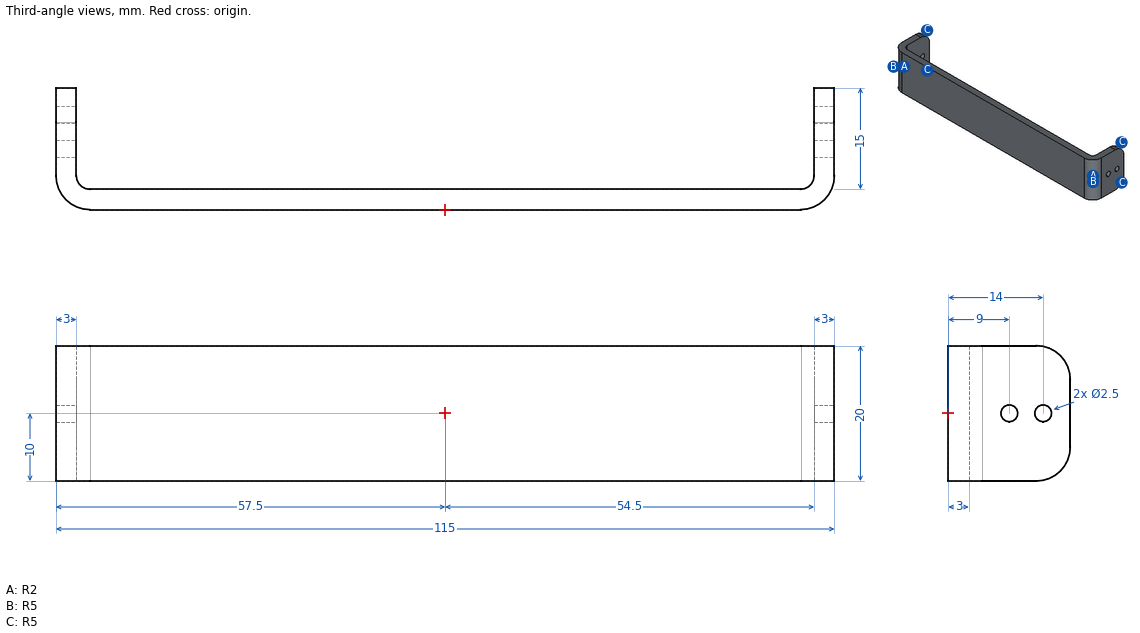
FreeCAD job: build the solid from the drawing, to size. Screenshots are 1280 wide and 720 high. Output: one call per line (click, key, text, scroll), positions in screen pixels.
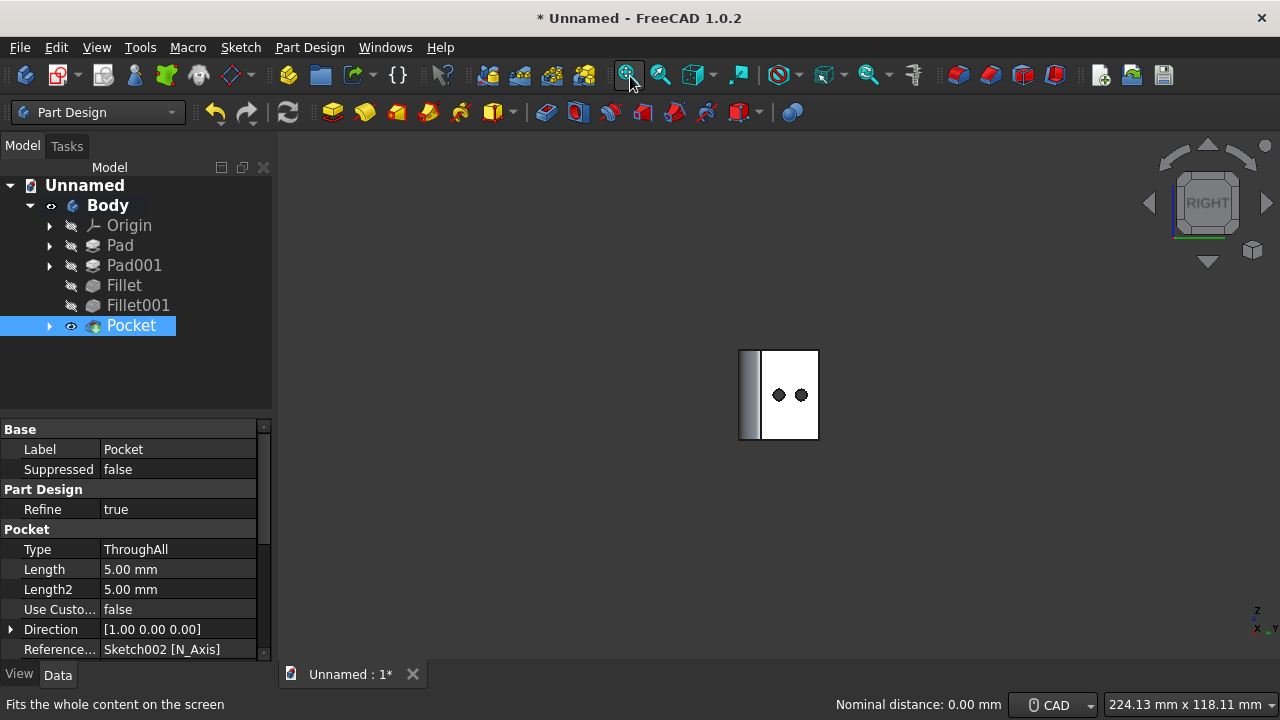
click(630, 76)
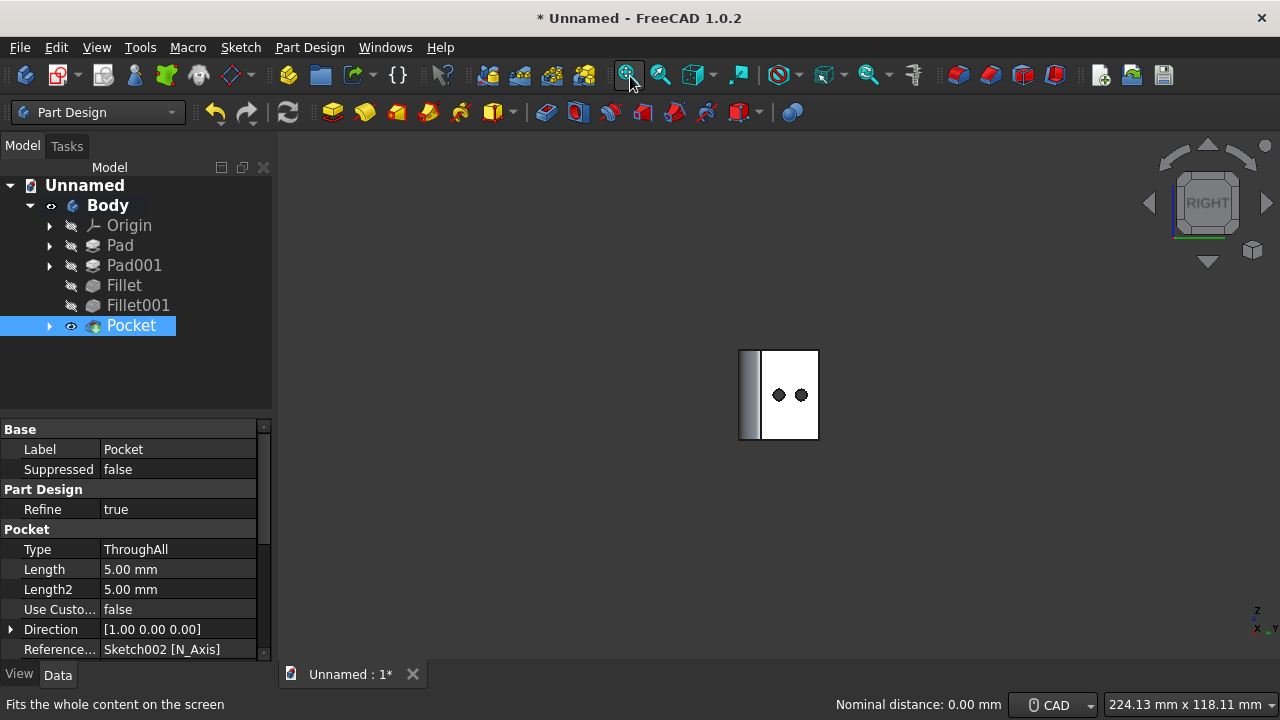
scroll(819, 439, up, 6)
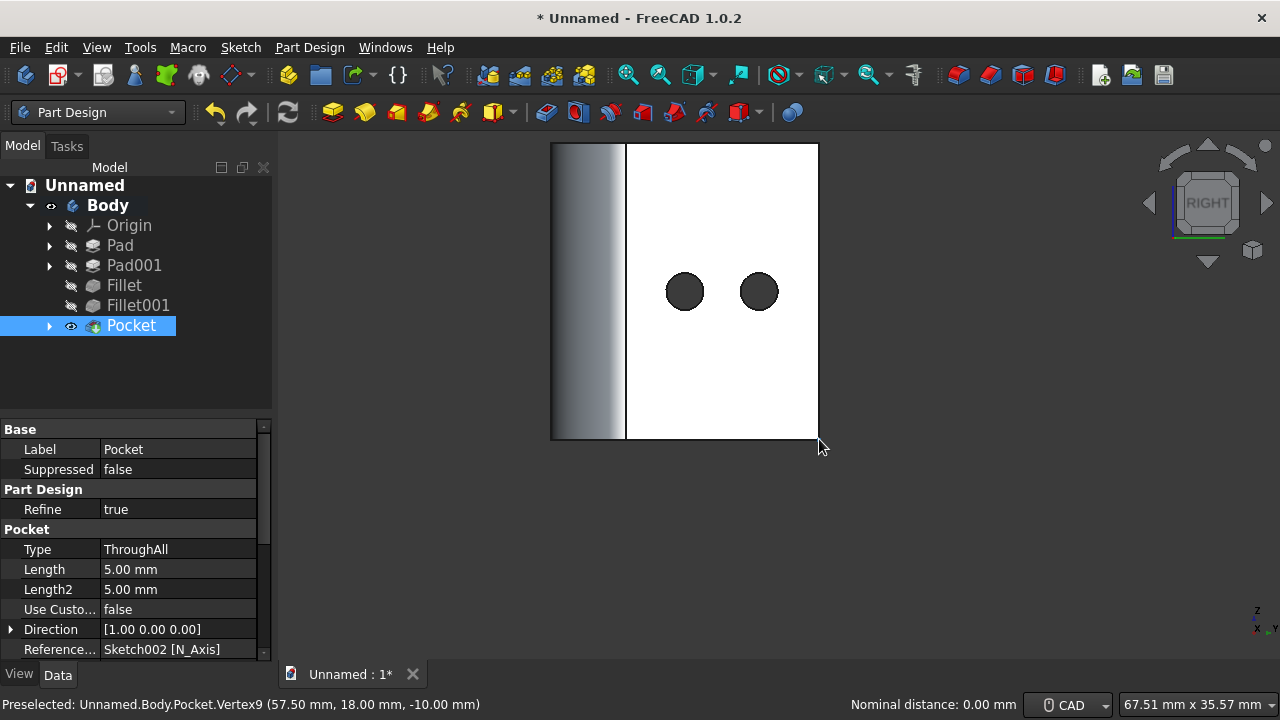
click(630, 76)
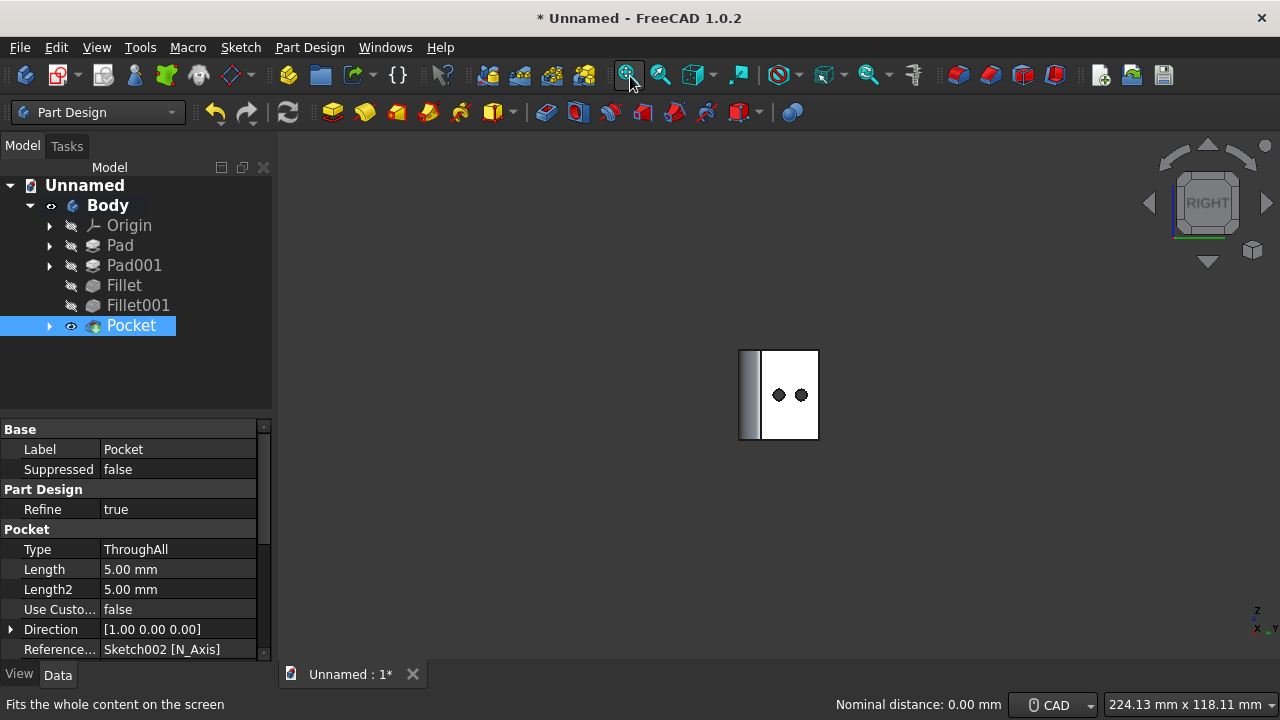
key(5)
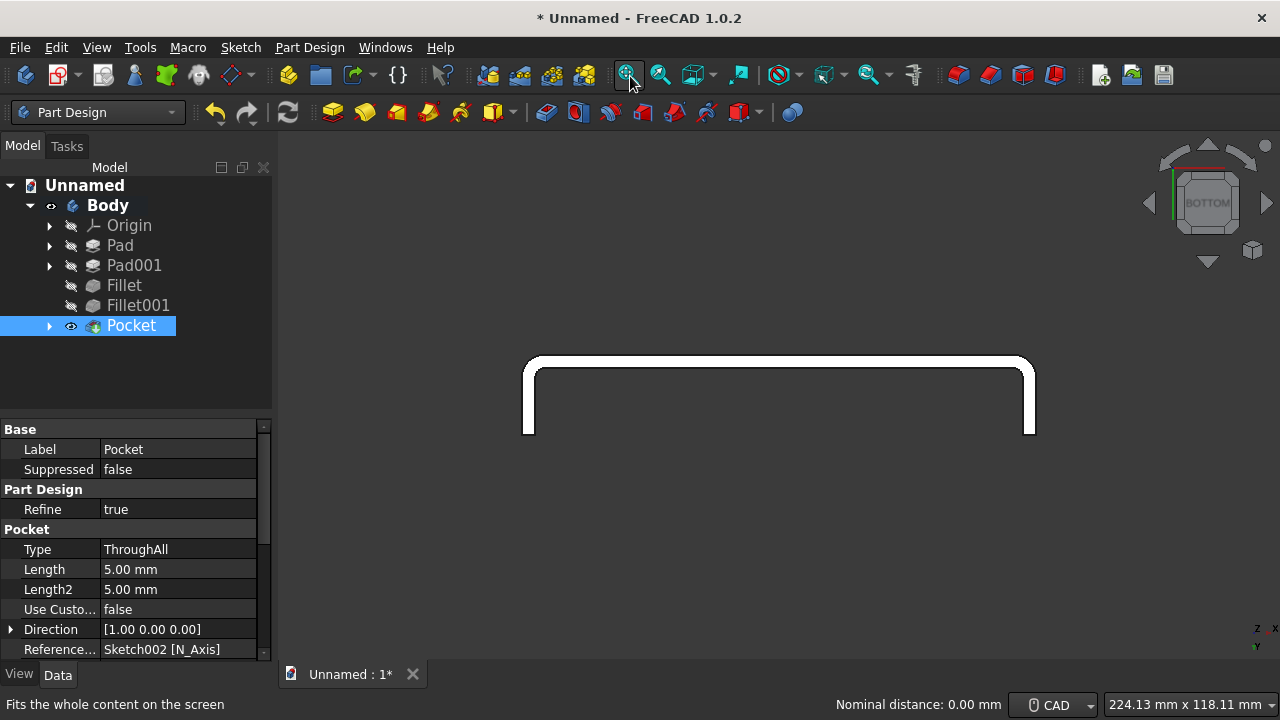
scroll(529, 434, up, 6)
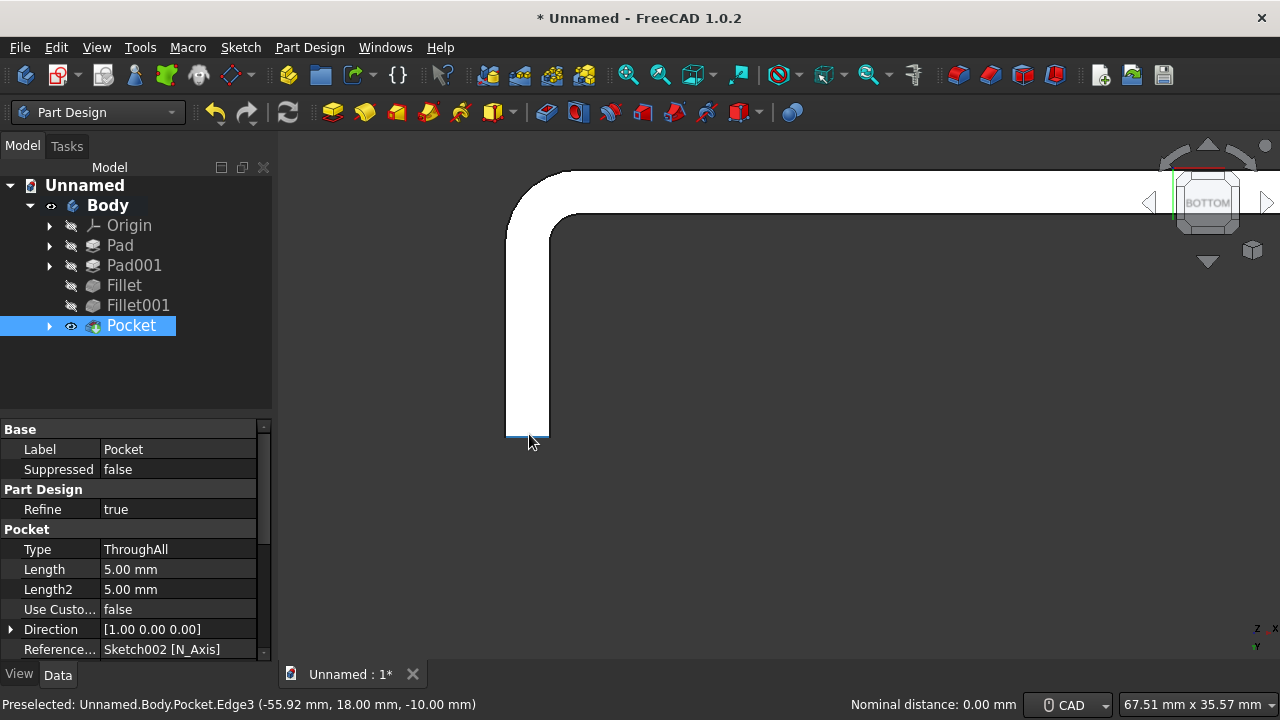
click(630, 76)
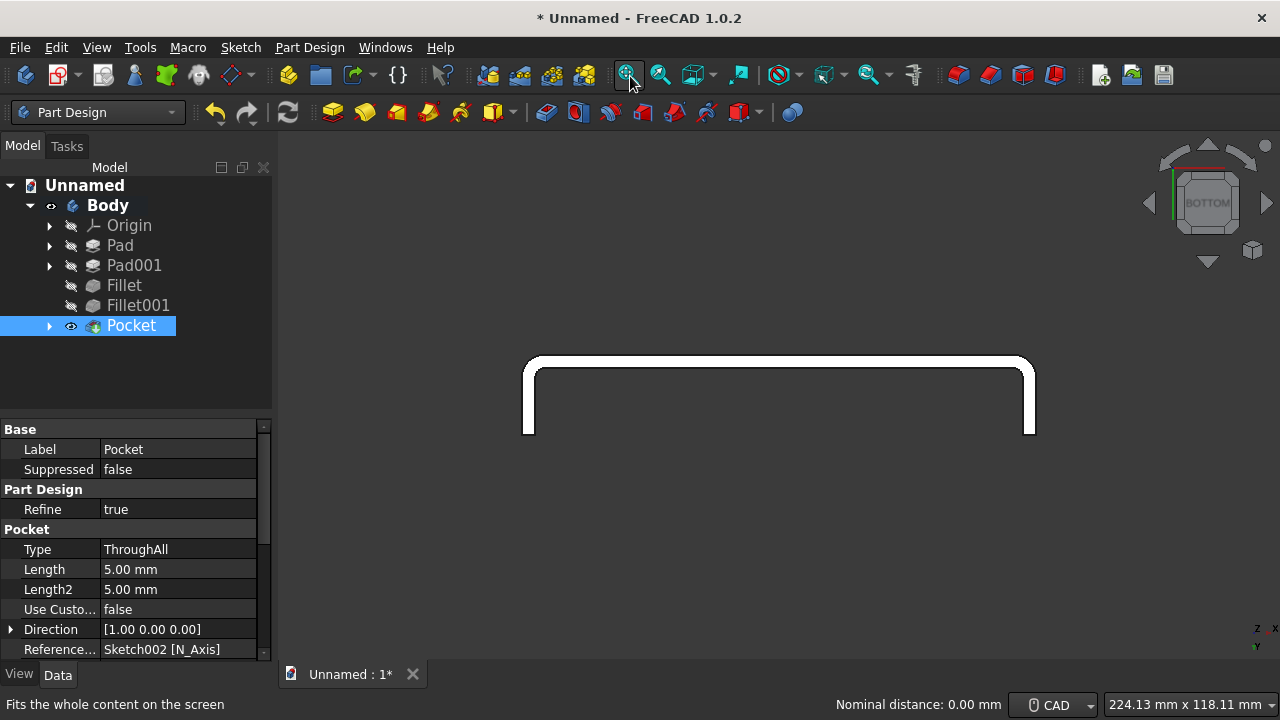
key(4)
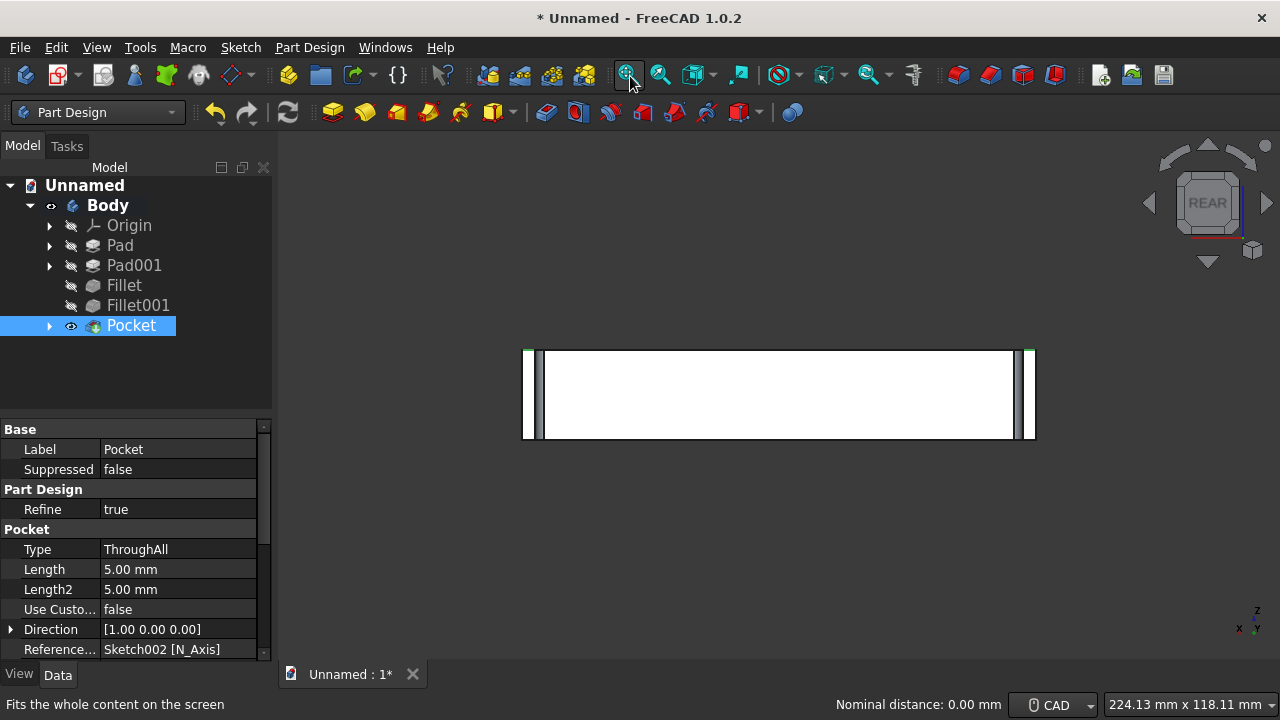
click(1029, 439, ctrl)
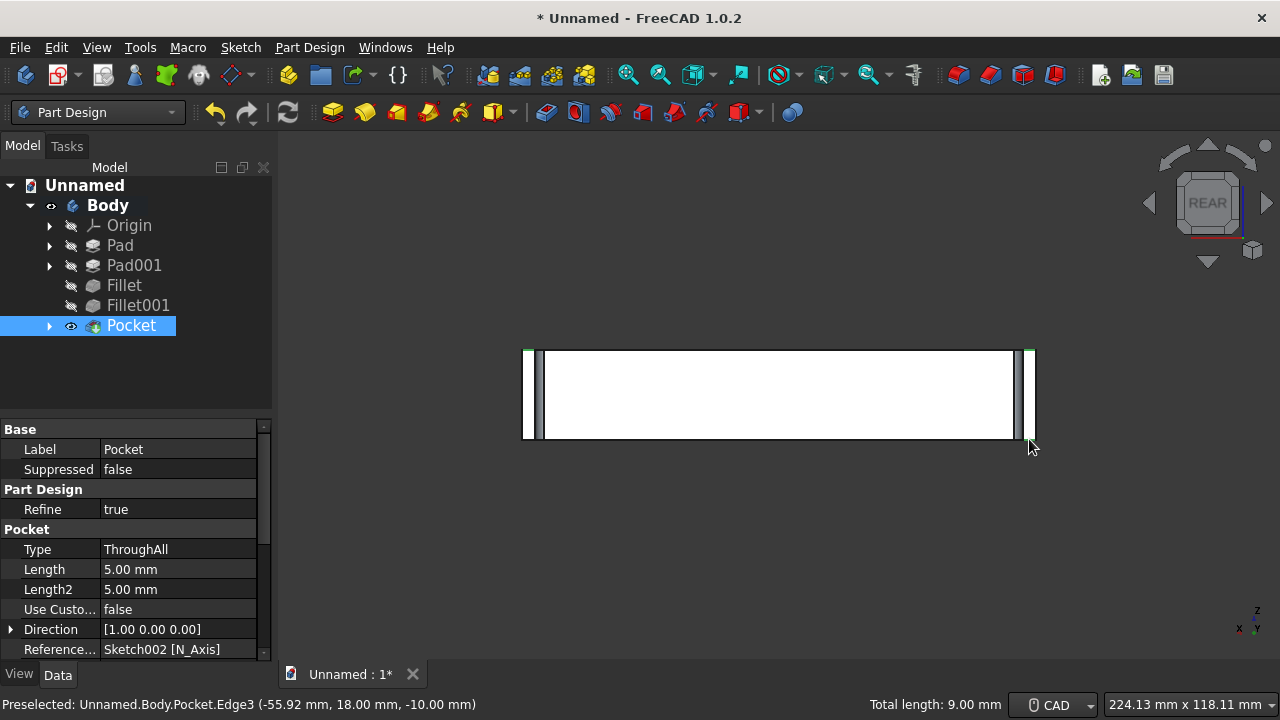
click(529, 439, ctrl)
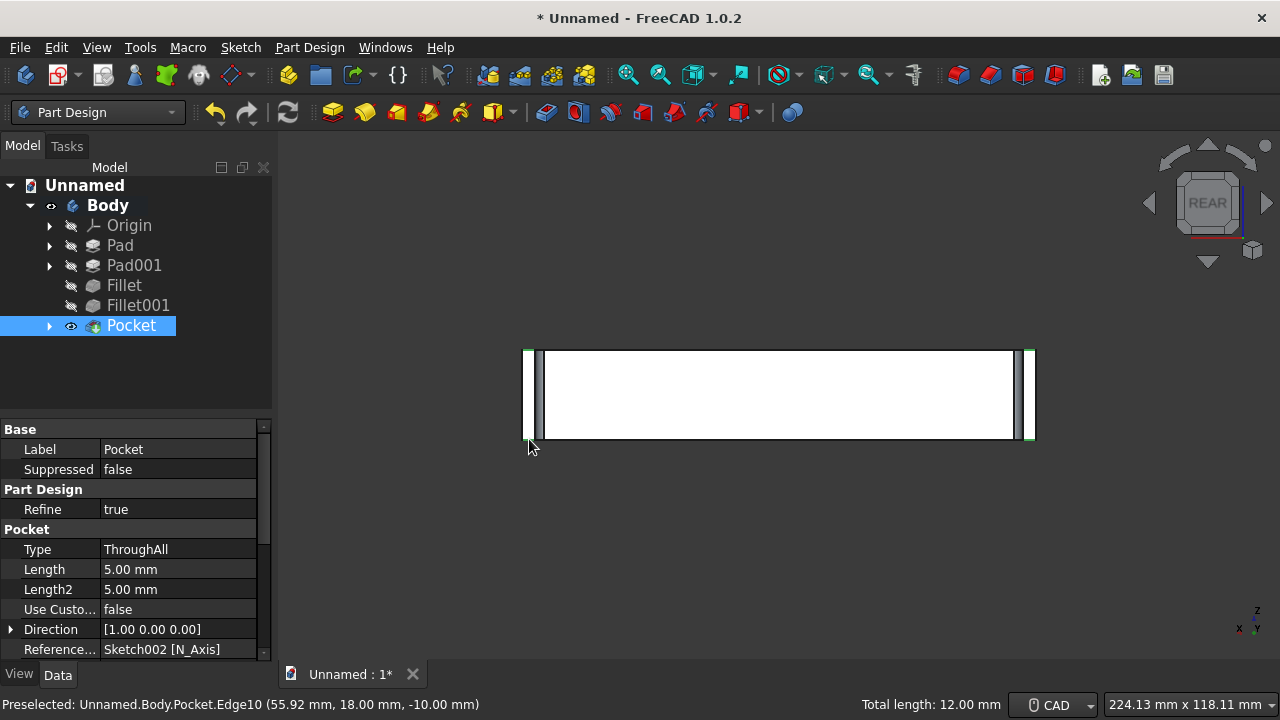
click(960, 76)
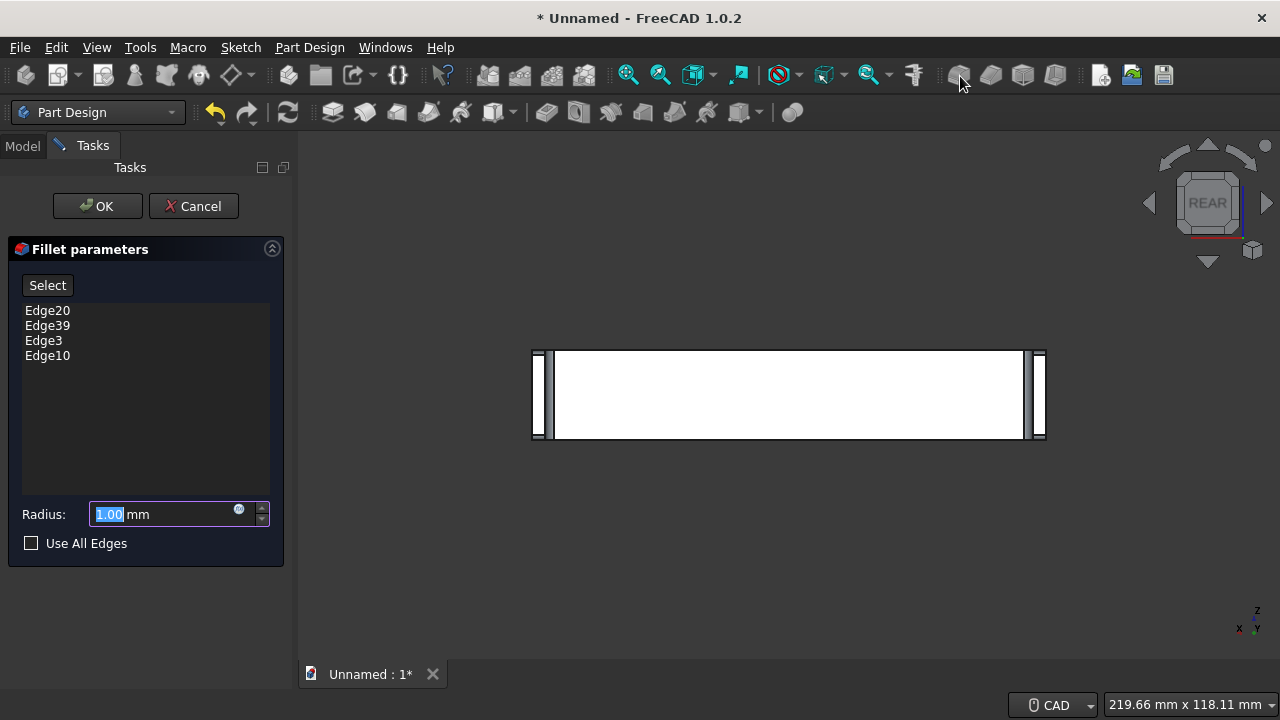
text(5)
key(Tab)